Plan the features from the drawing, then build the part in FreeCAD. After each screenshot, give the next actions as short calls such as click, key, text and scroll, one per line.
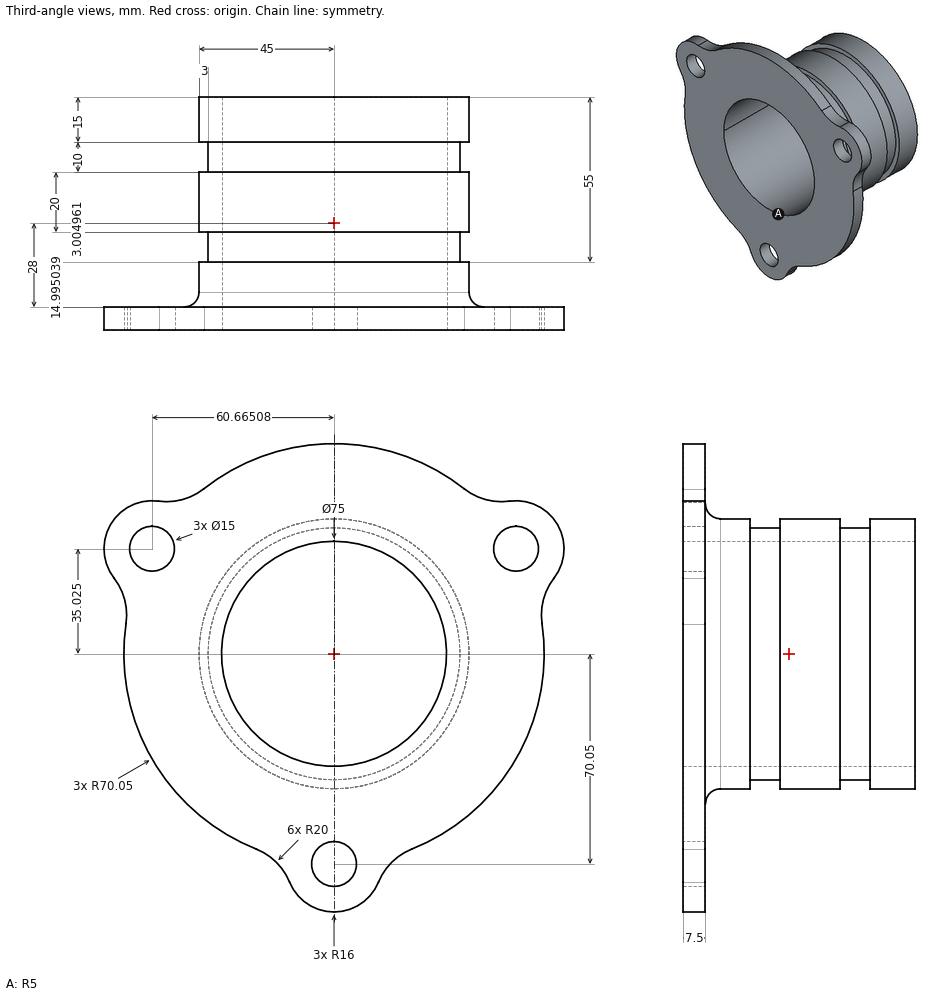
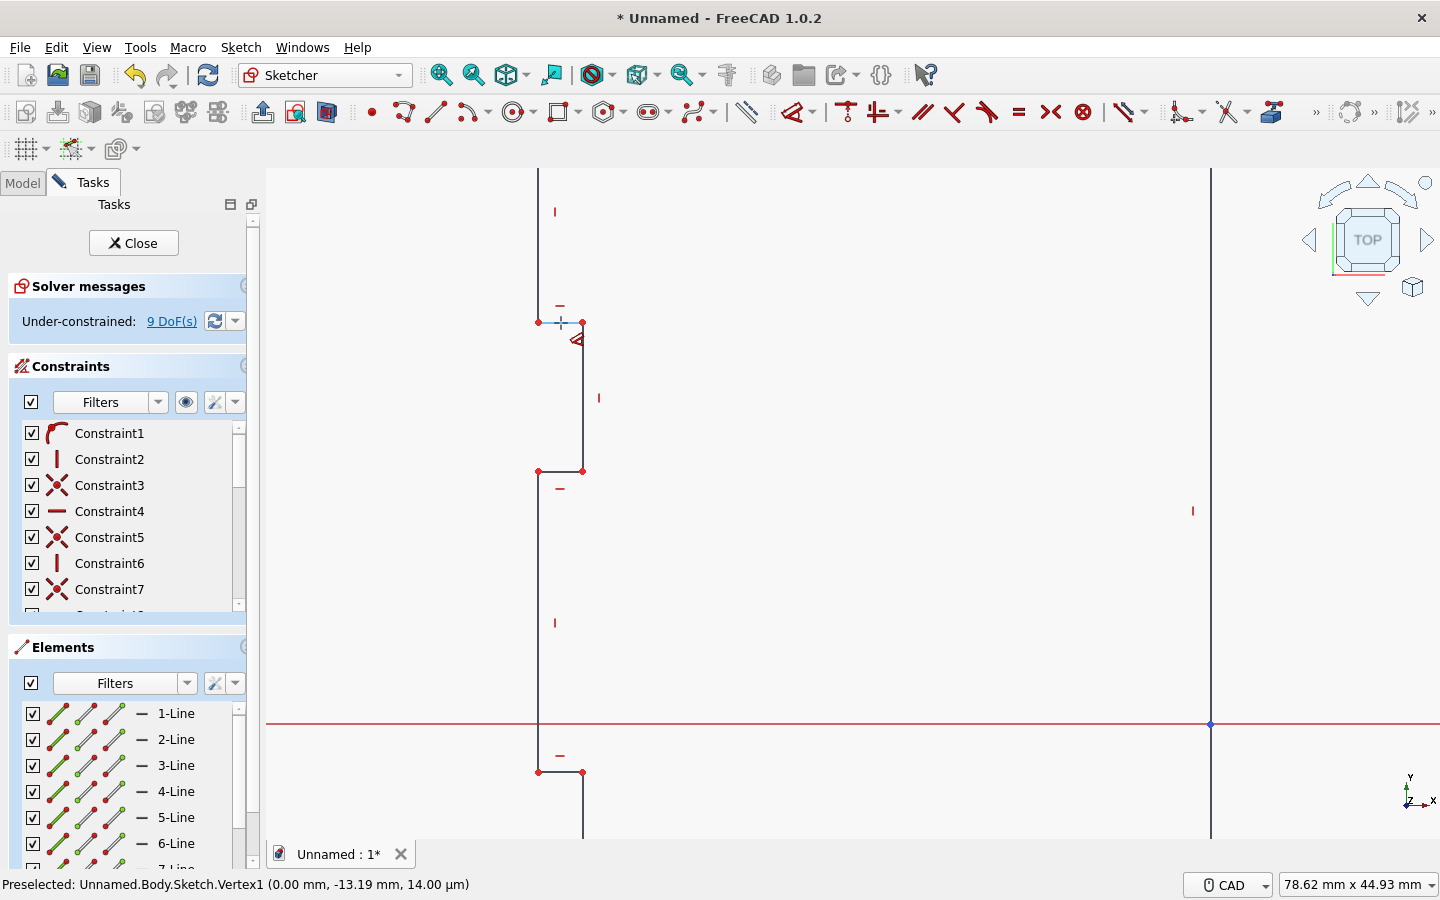
click(561, 323)
click(561, 289)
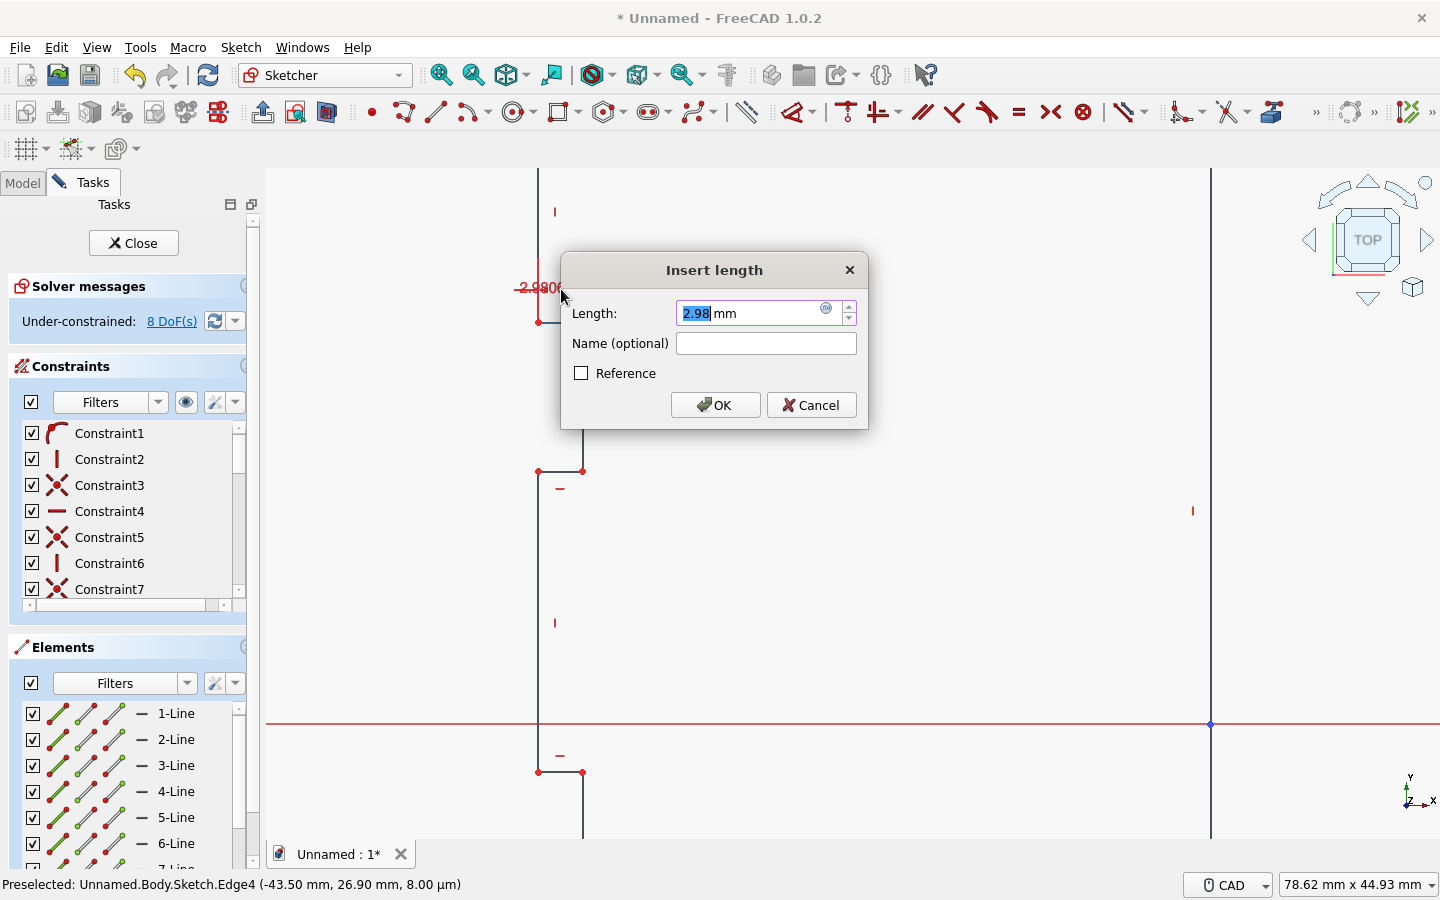
text(3)
key(Return)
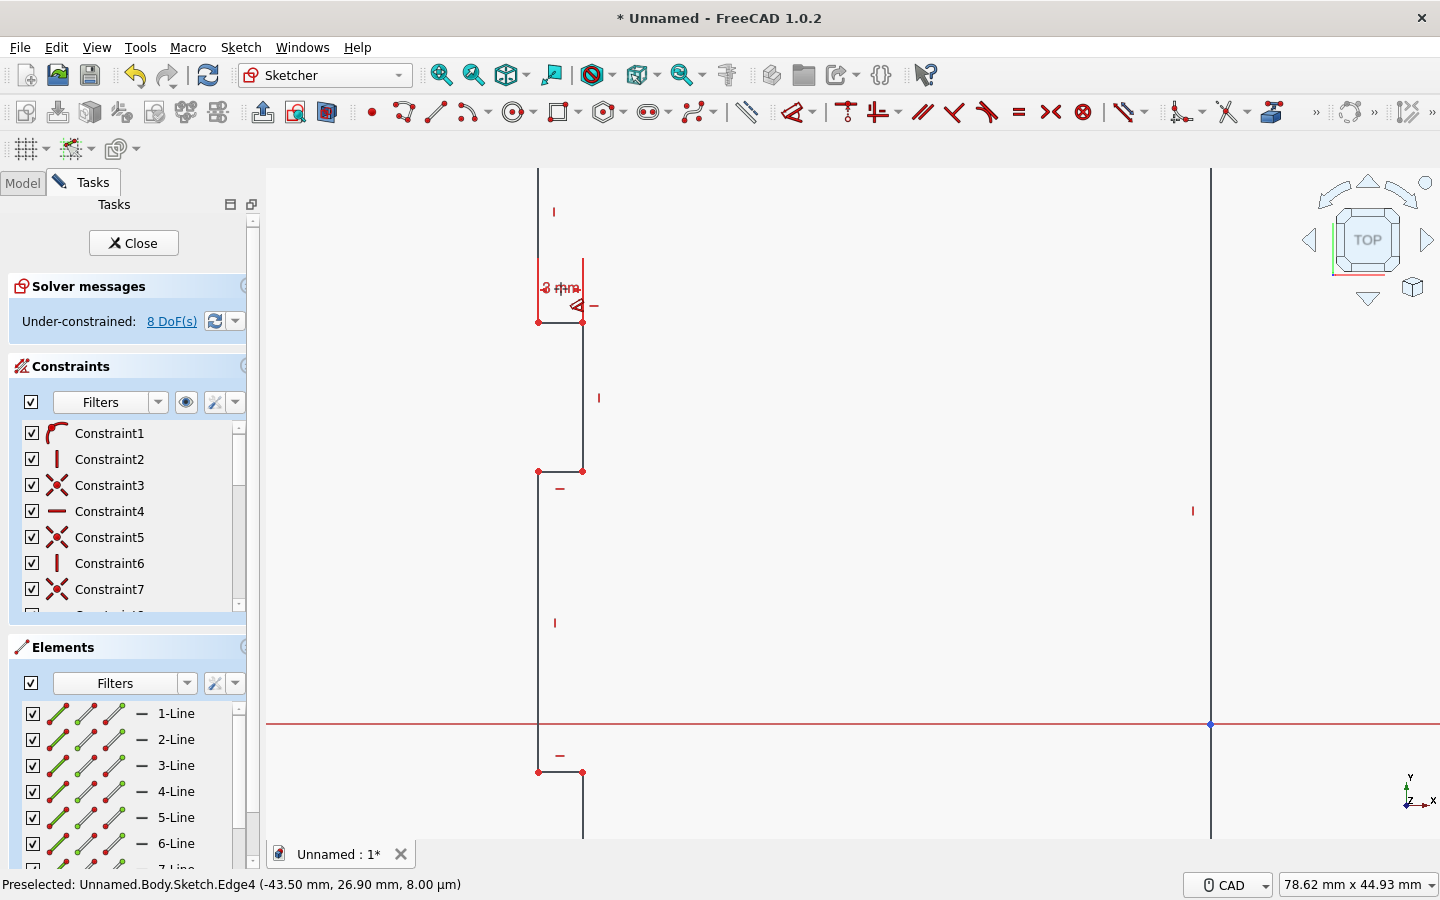
click(570, 472)
click(561, 438)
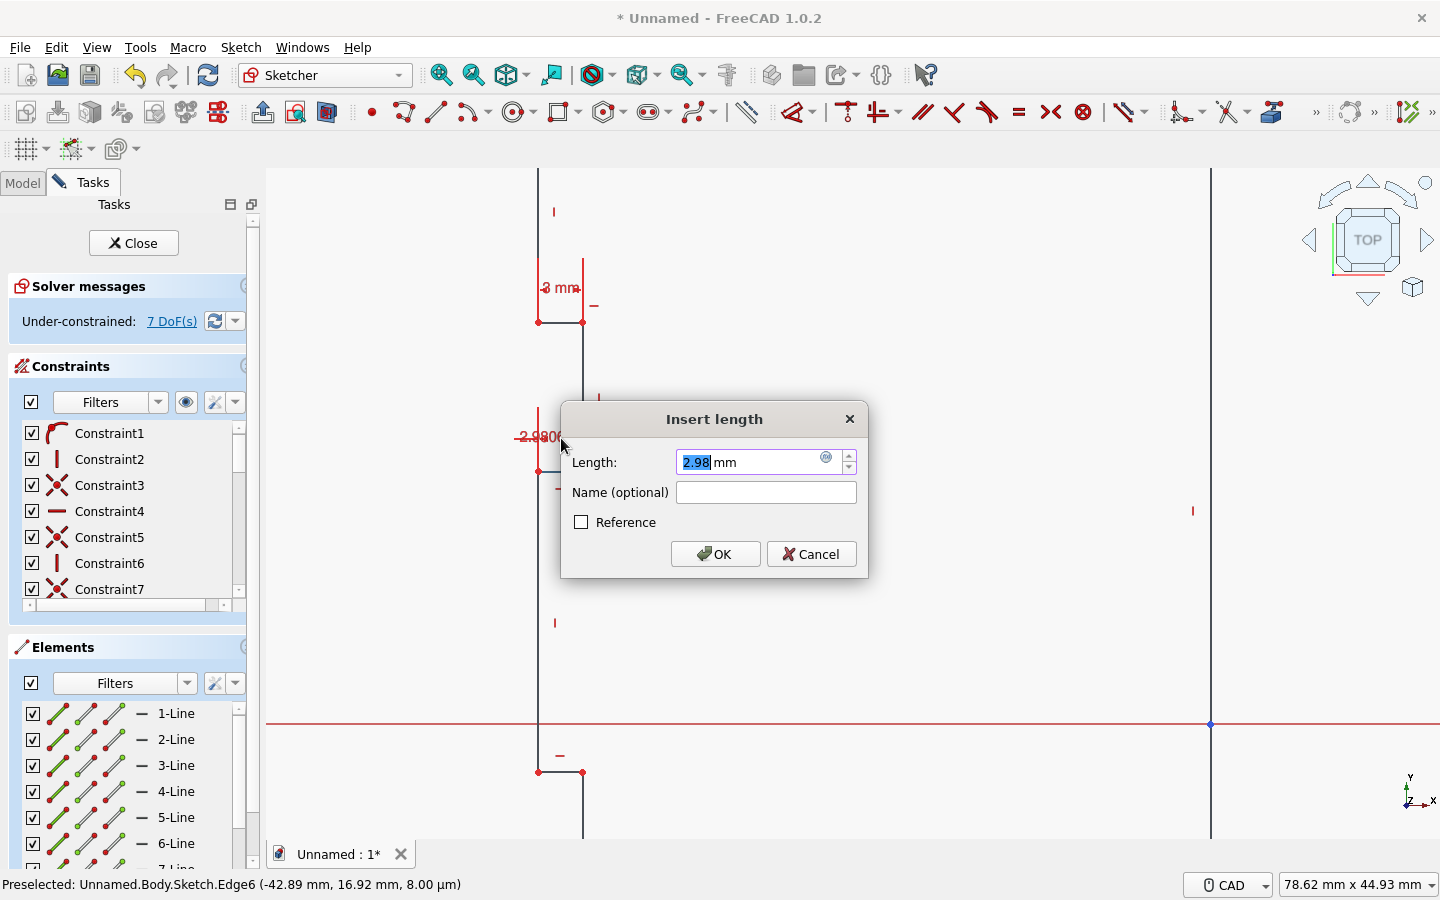
text(3)
key(Return)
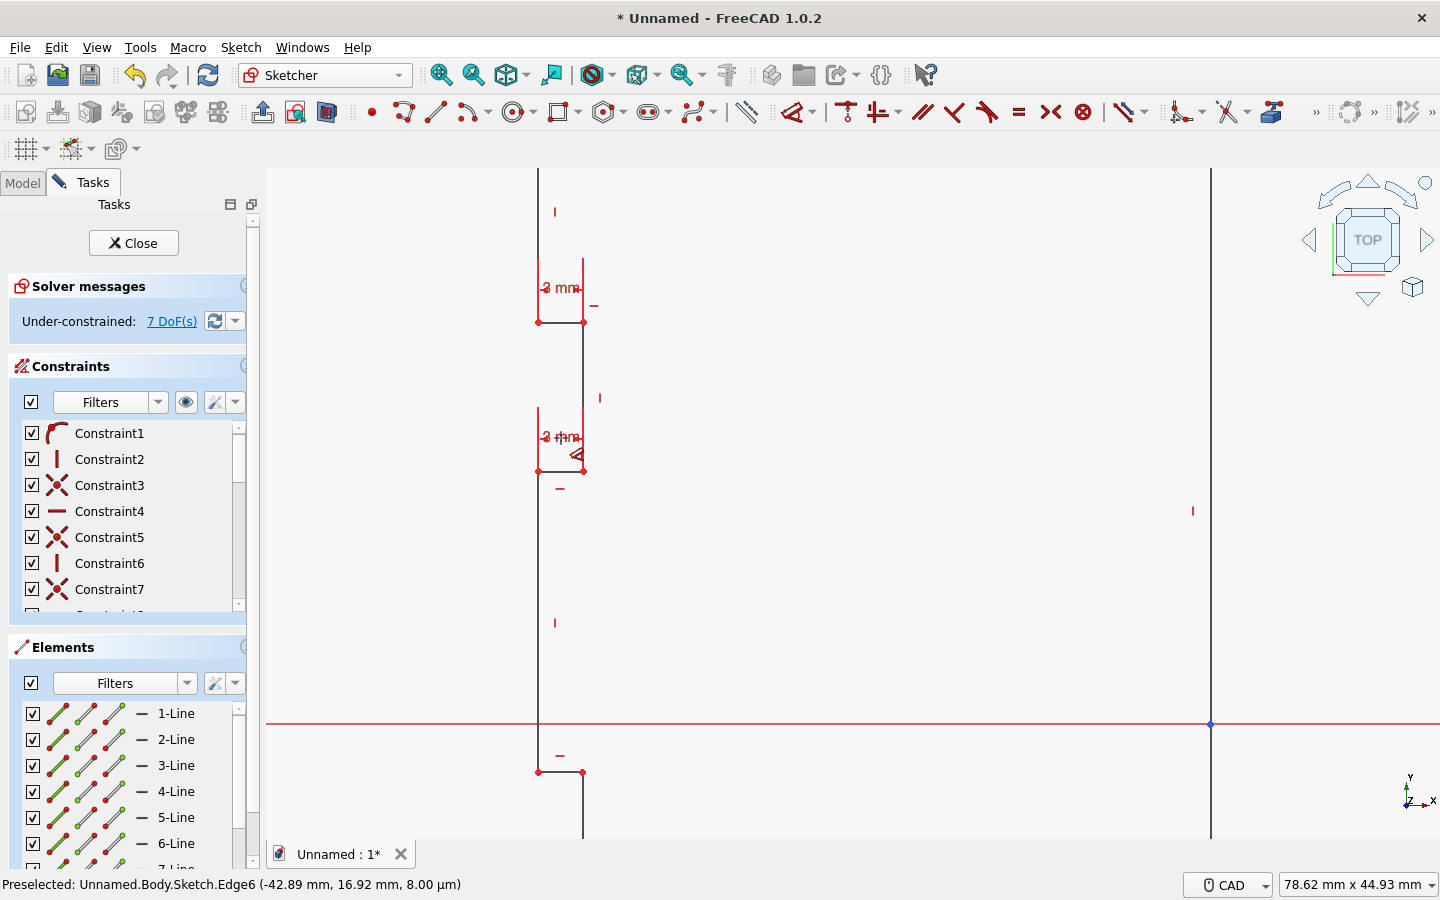
click(552, 772)
click(561, 806)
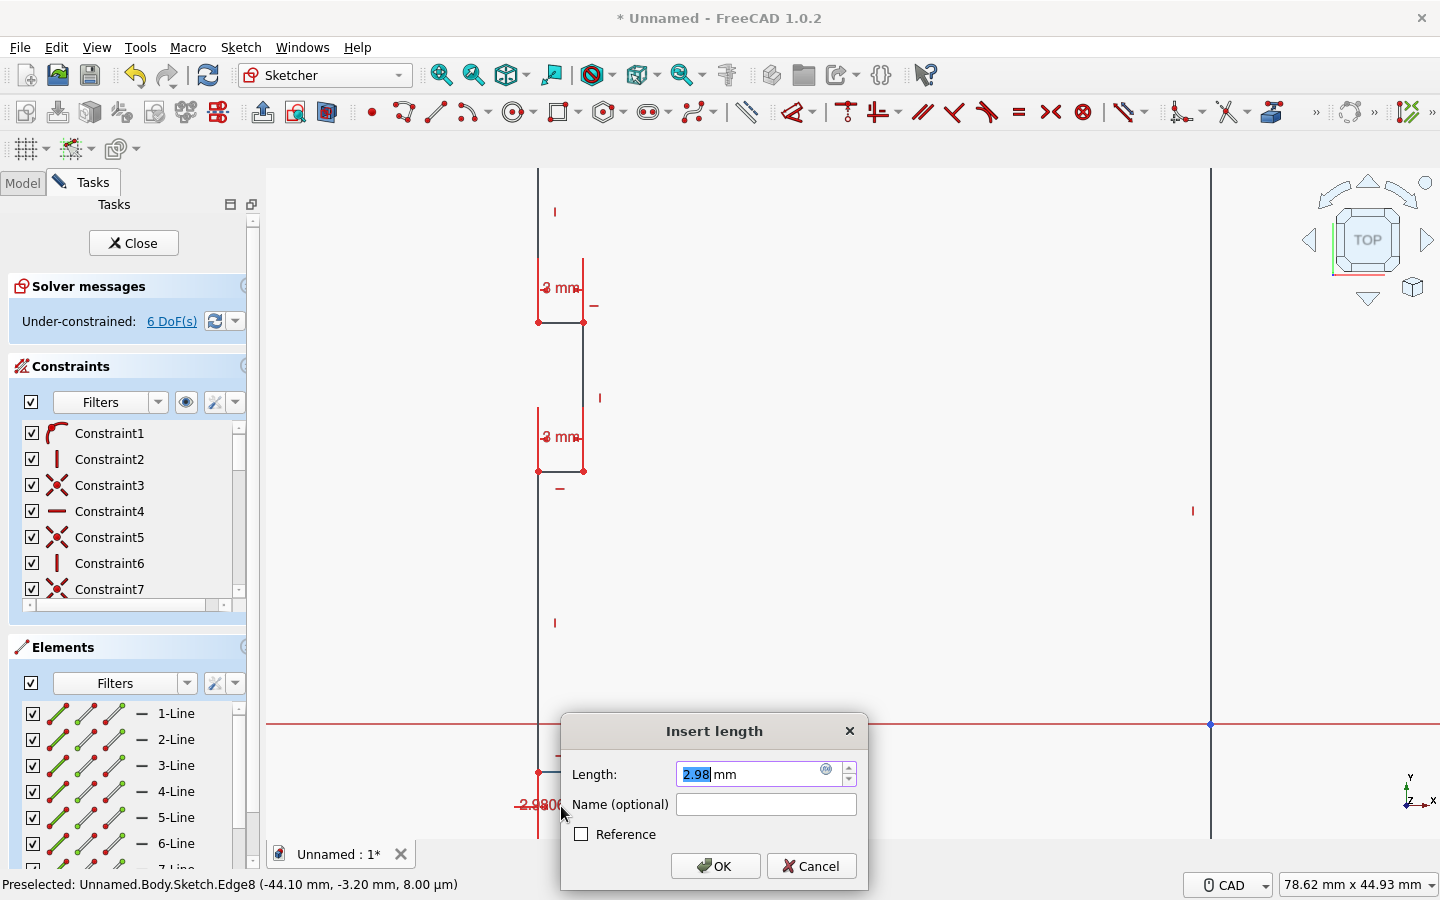
text(3)
key(Return)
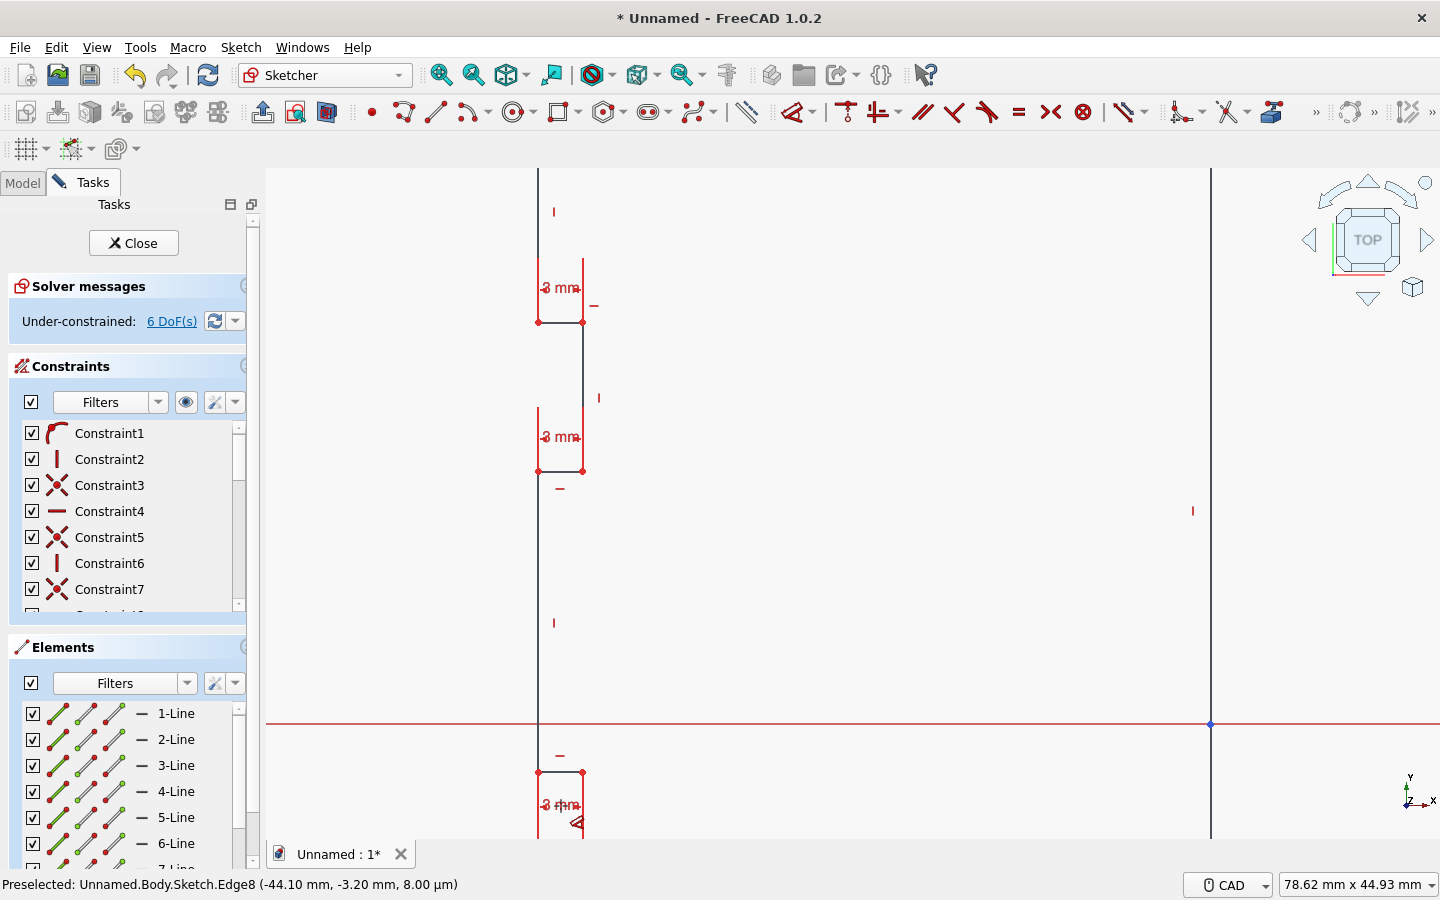
click(1211, 675)
click(1245, 504)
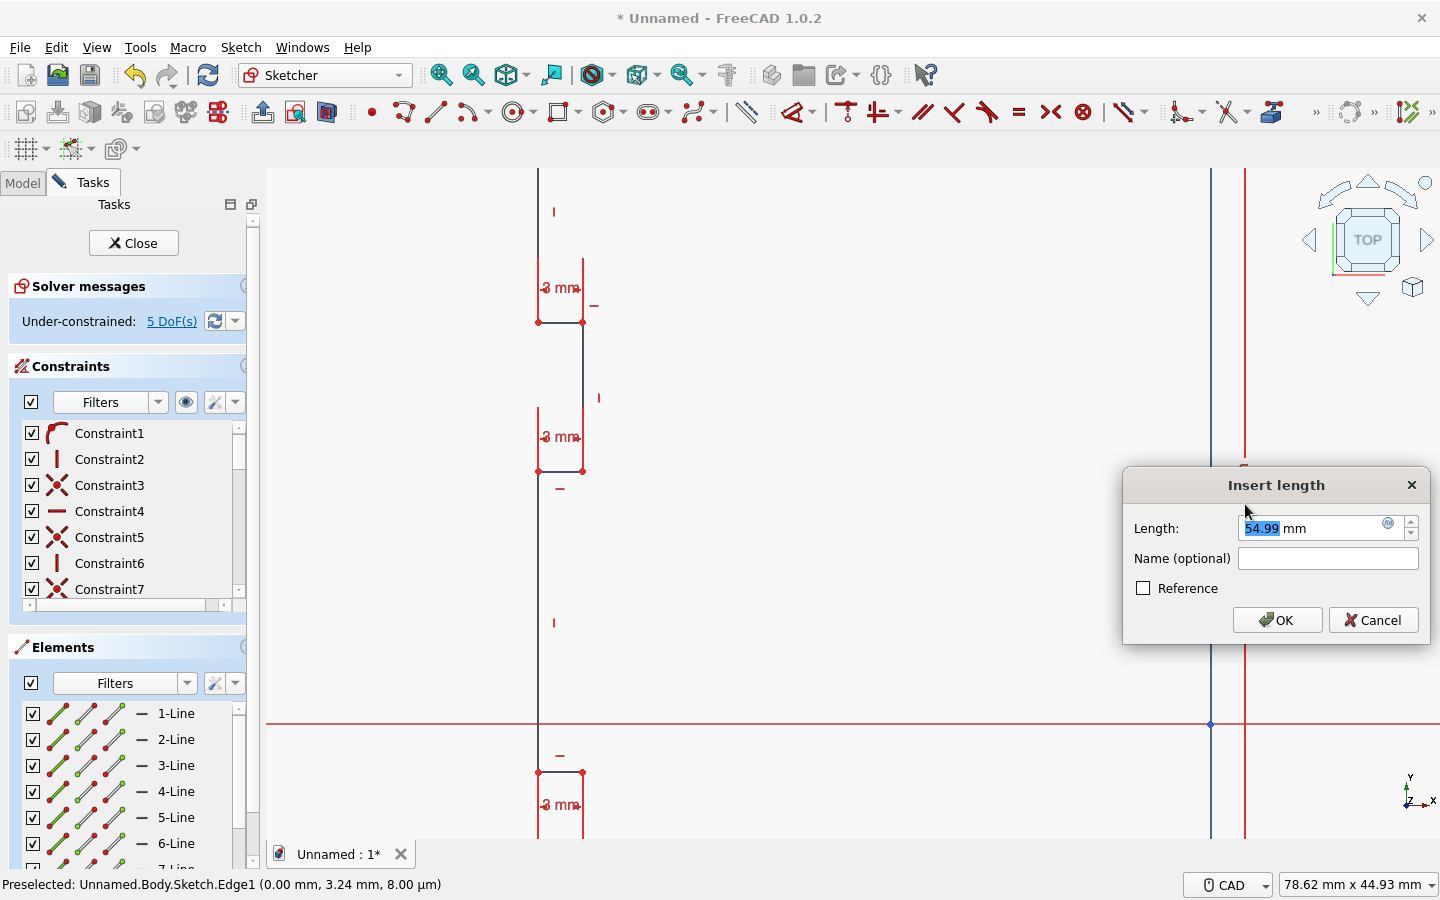
text(55)
key(Return)